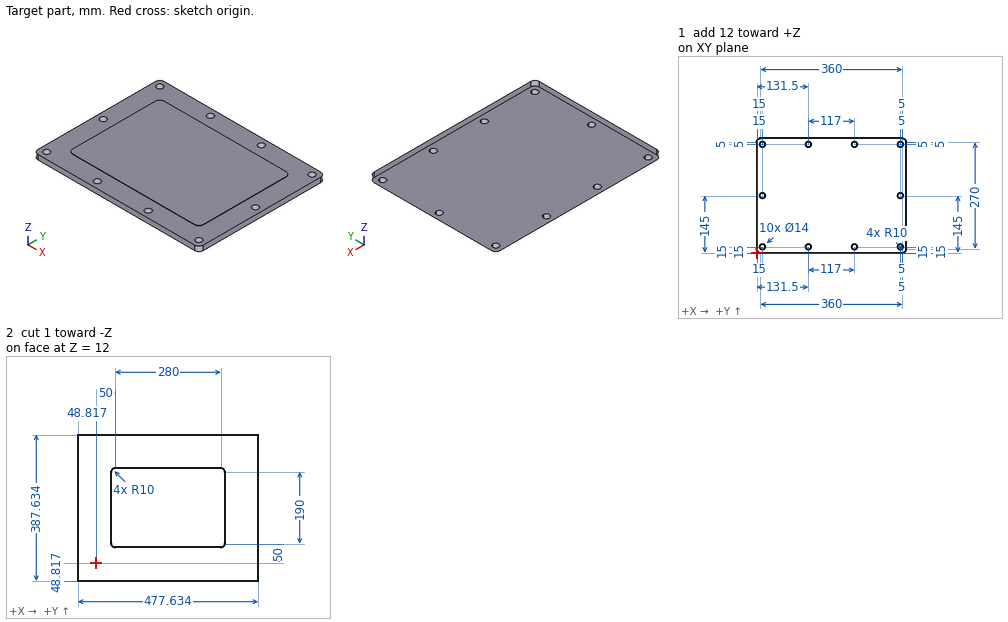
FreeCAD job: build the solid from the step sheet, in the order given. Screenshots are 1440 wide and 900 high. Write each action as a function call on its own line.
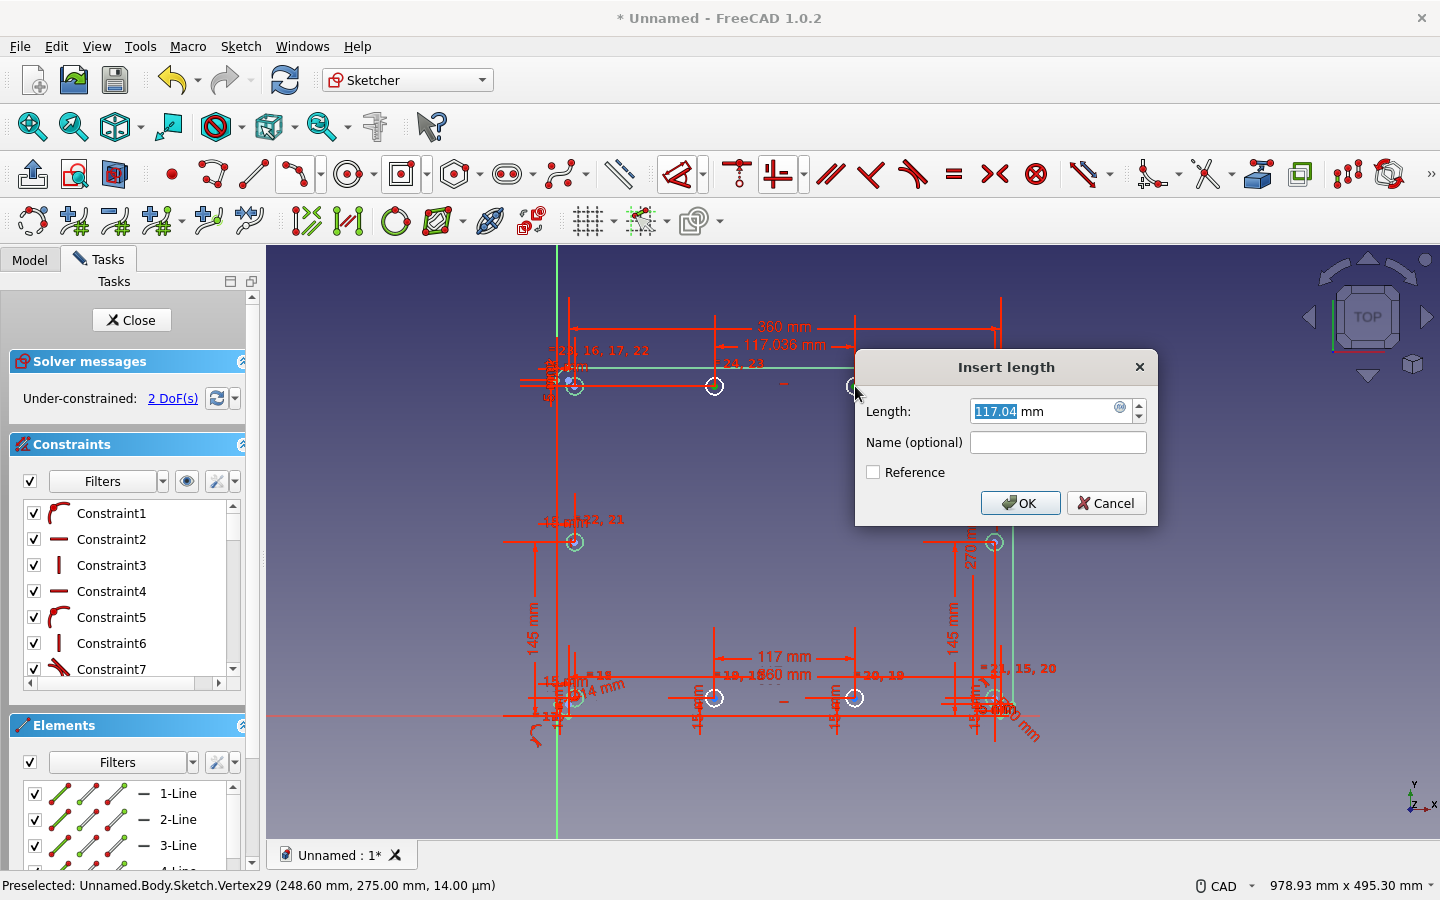
text(117)
key(Return)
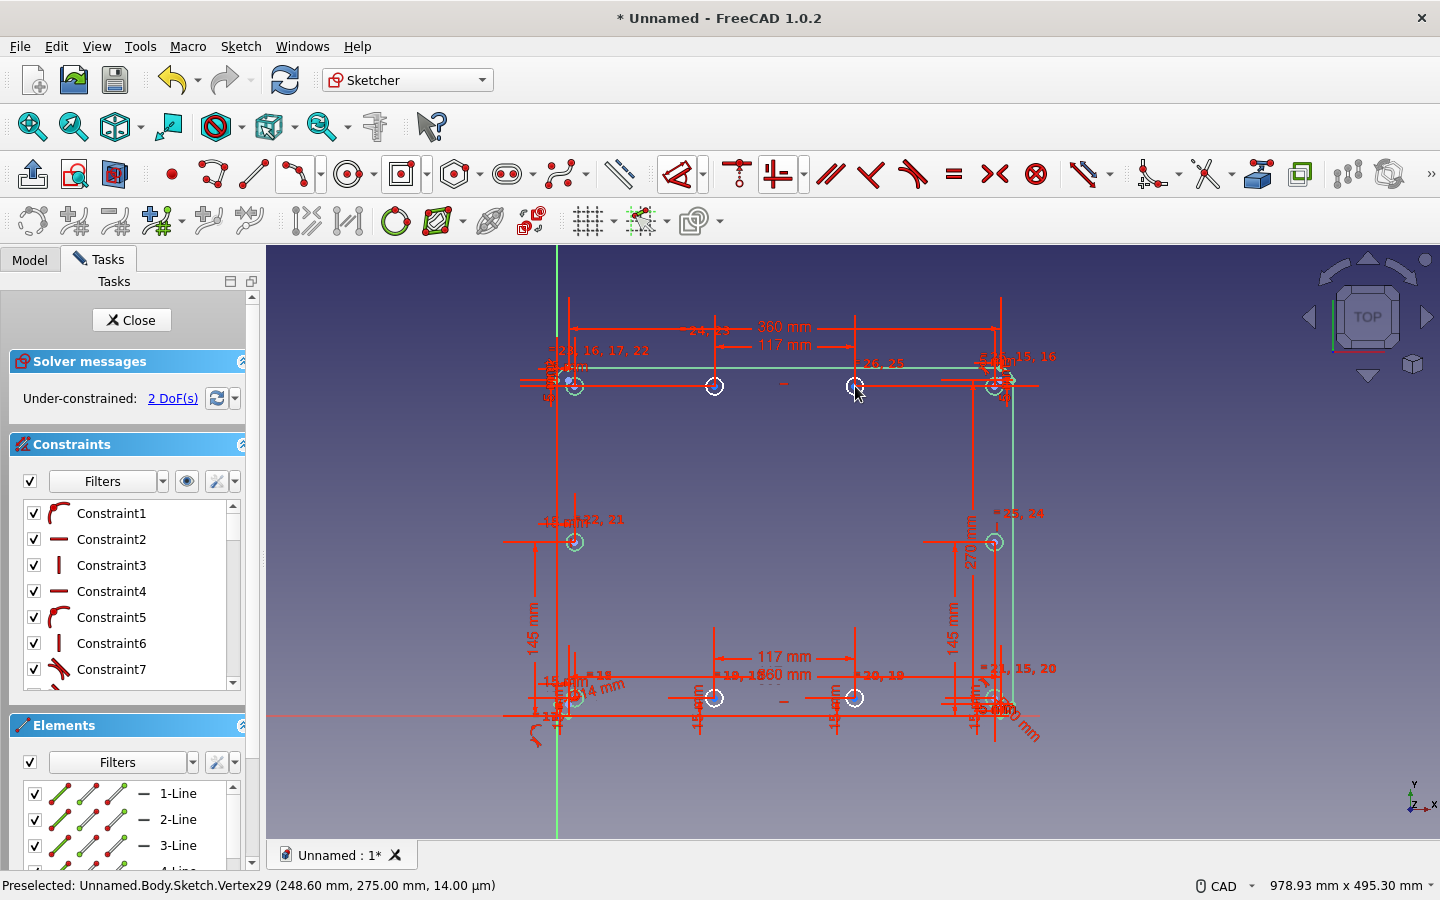
click(714, 698)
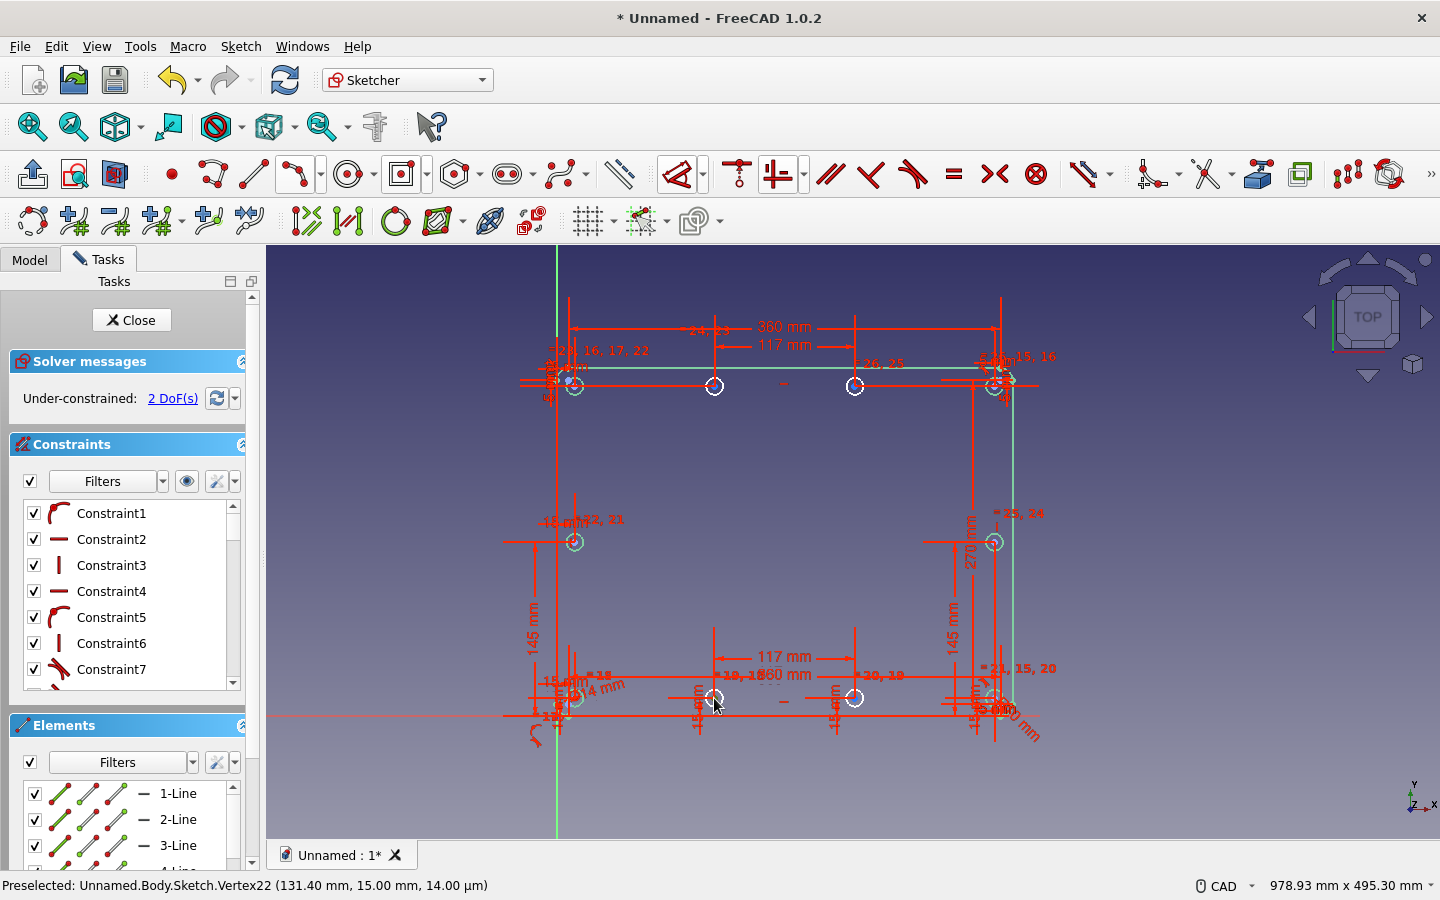
click(702, 174)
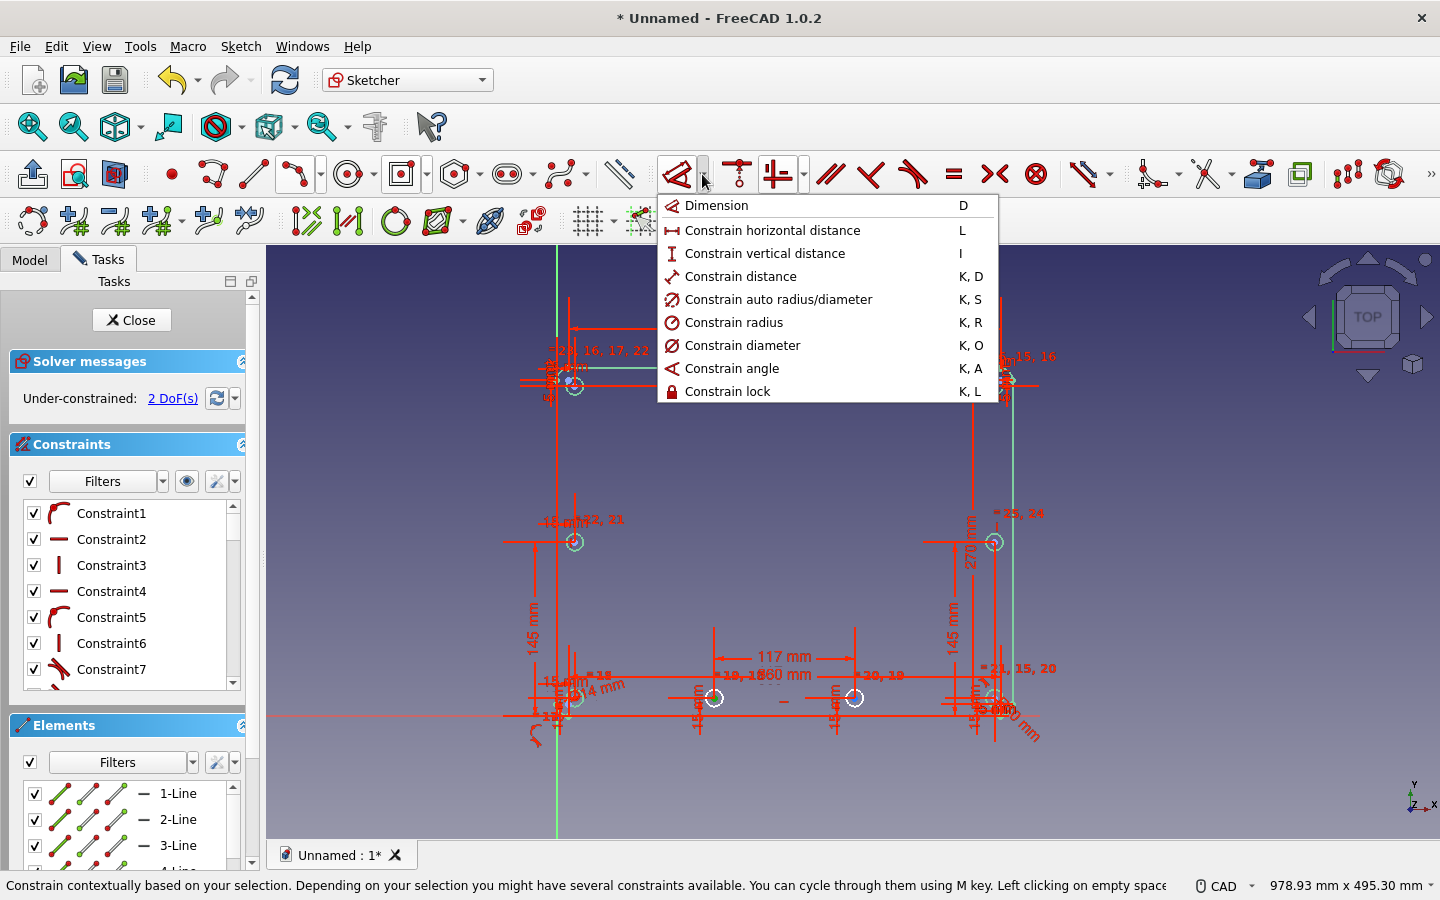
click(828, 230)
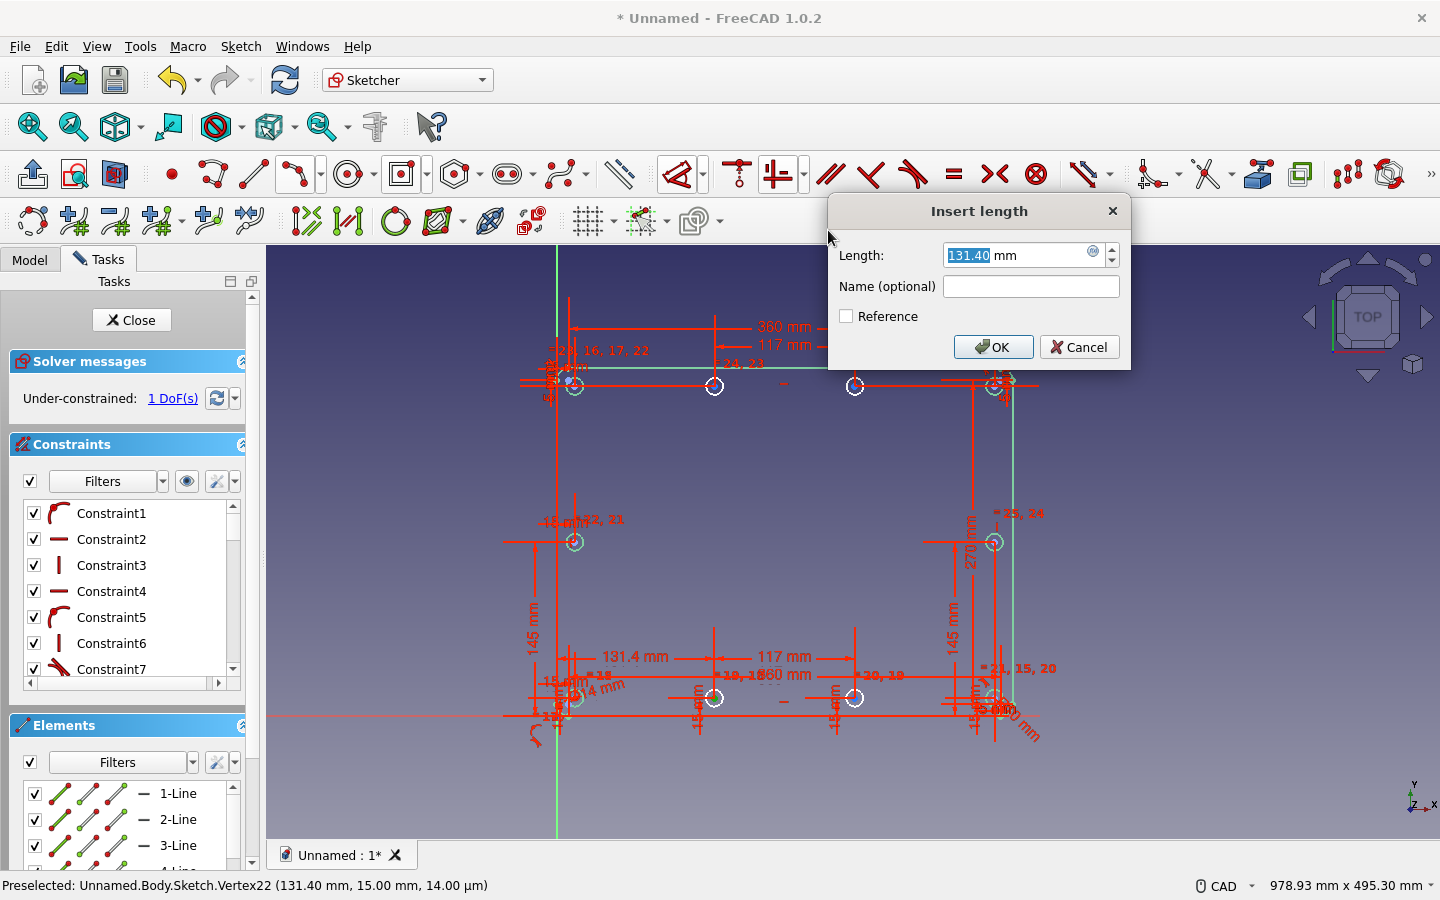
text(131.5)
key(Return)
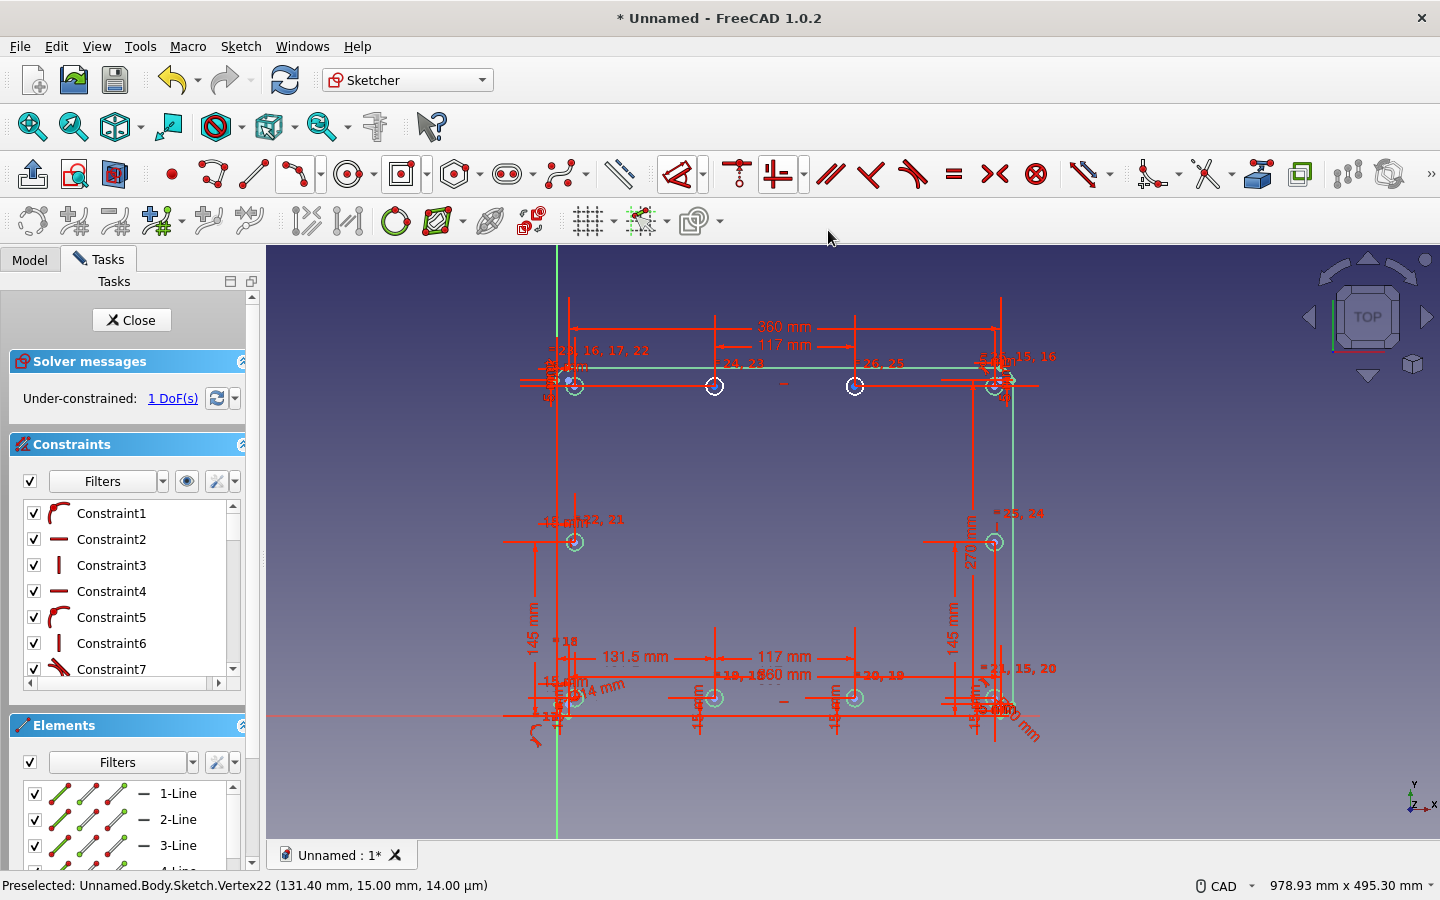
click(715, 386)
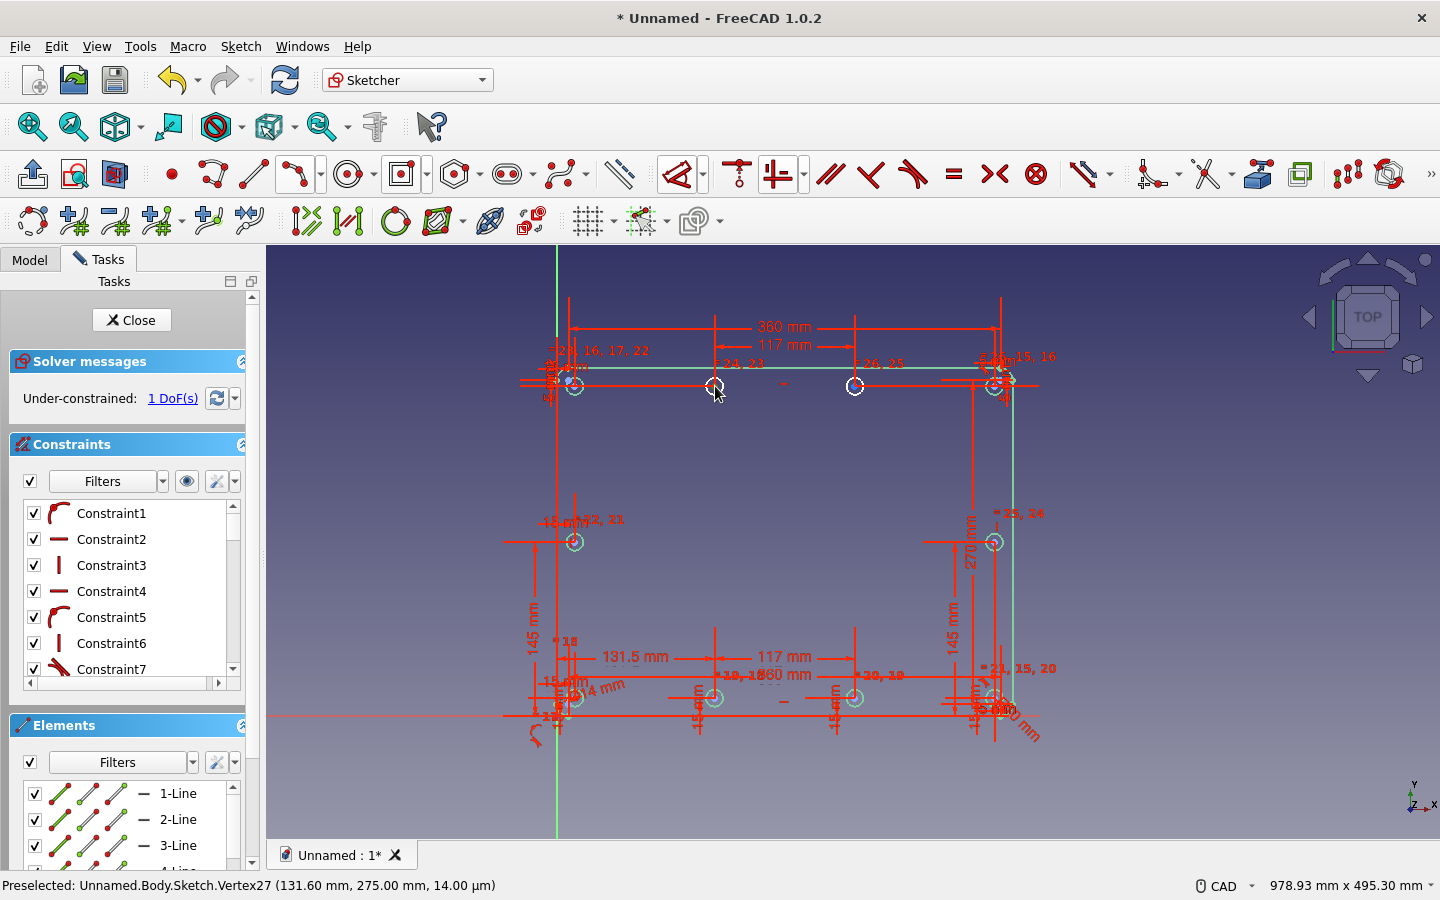
click(702, 174)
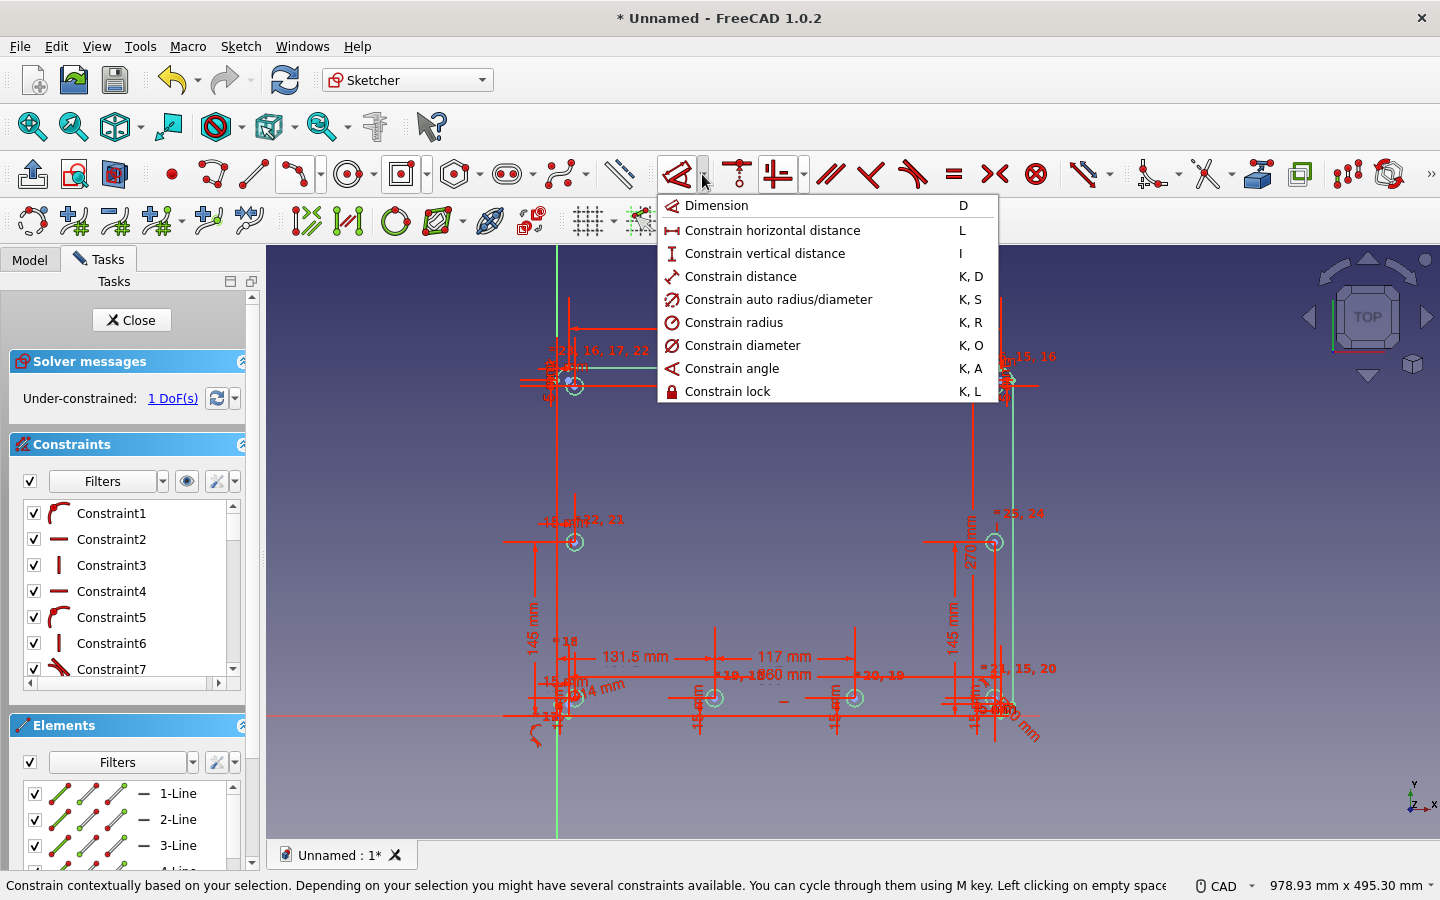
click(828, 230)